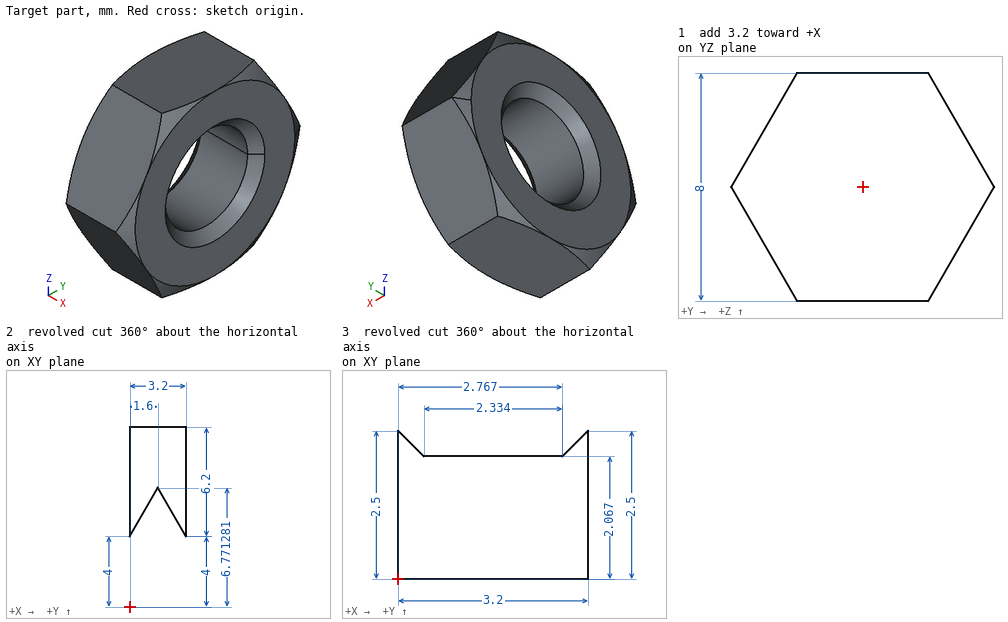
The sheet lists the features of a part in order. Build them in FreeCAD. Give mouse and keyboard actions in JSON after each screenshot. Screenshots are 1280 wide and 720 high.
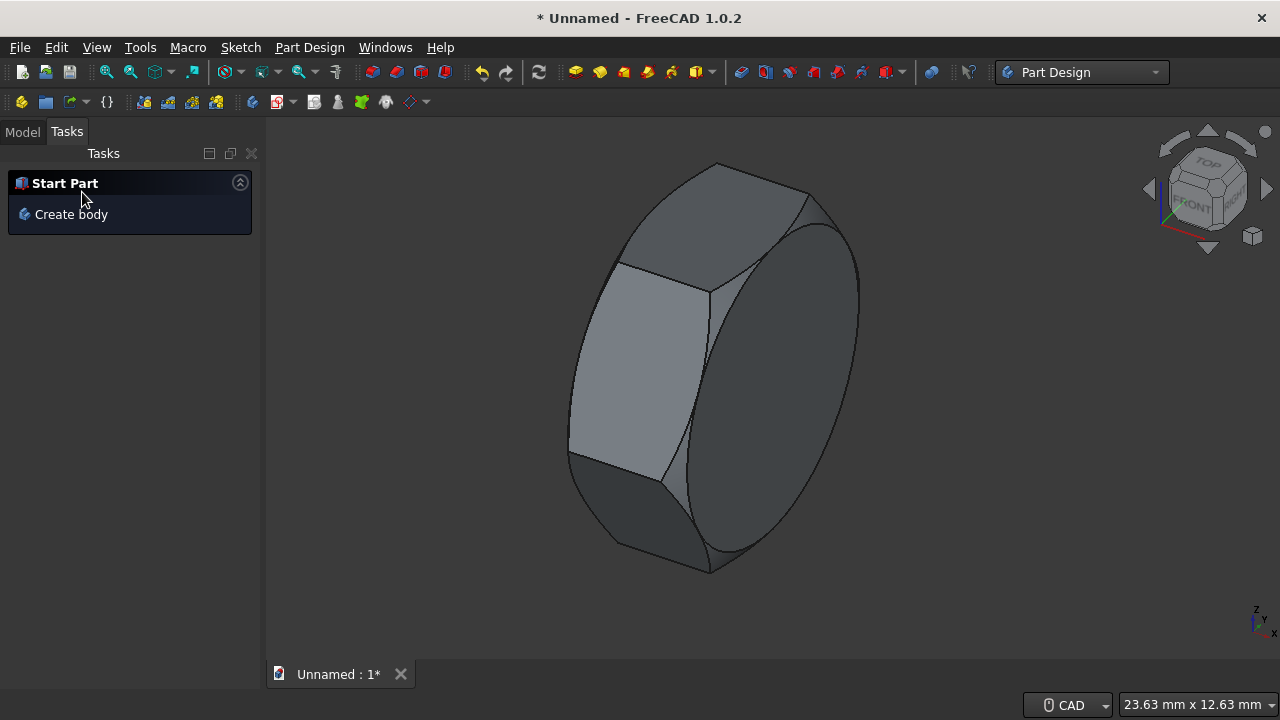
{"action": "key", "text": "v f"}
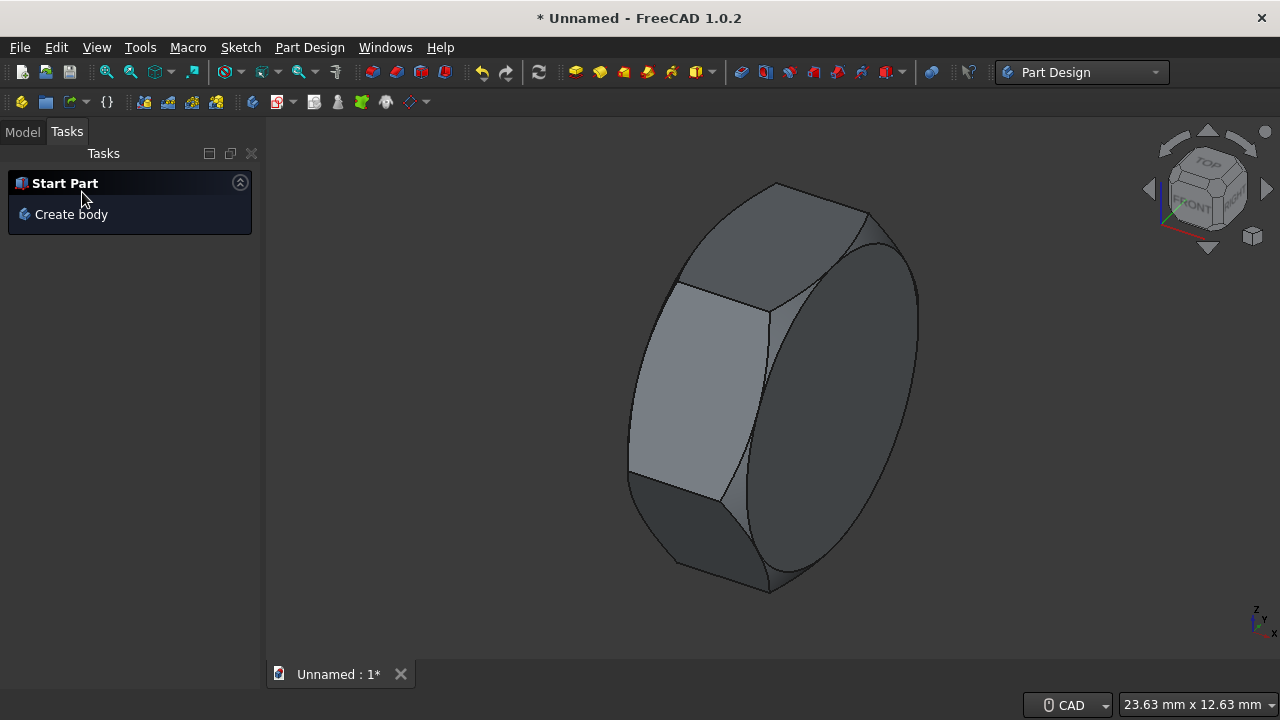
{"action": "left_click", "coordinate": [278, 102]}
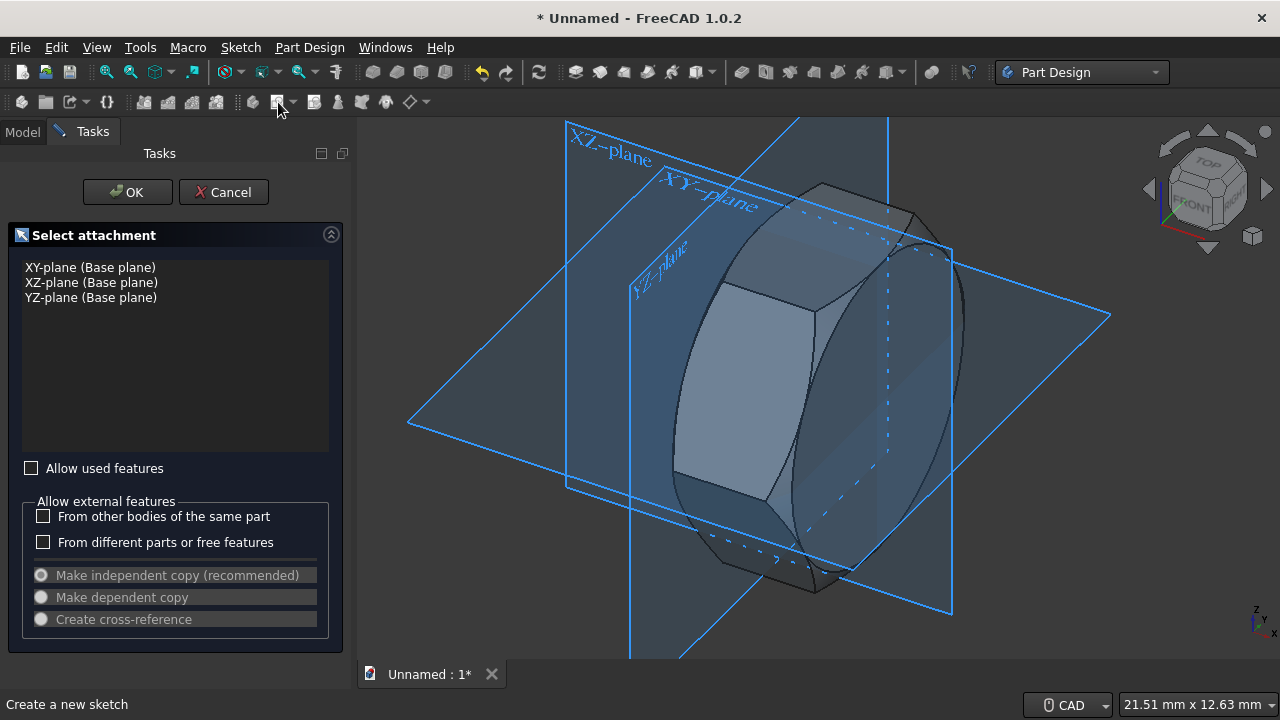
{"action": "left_click", "coordinate": [82, 268]}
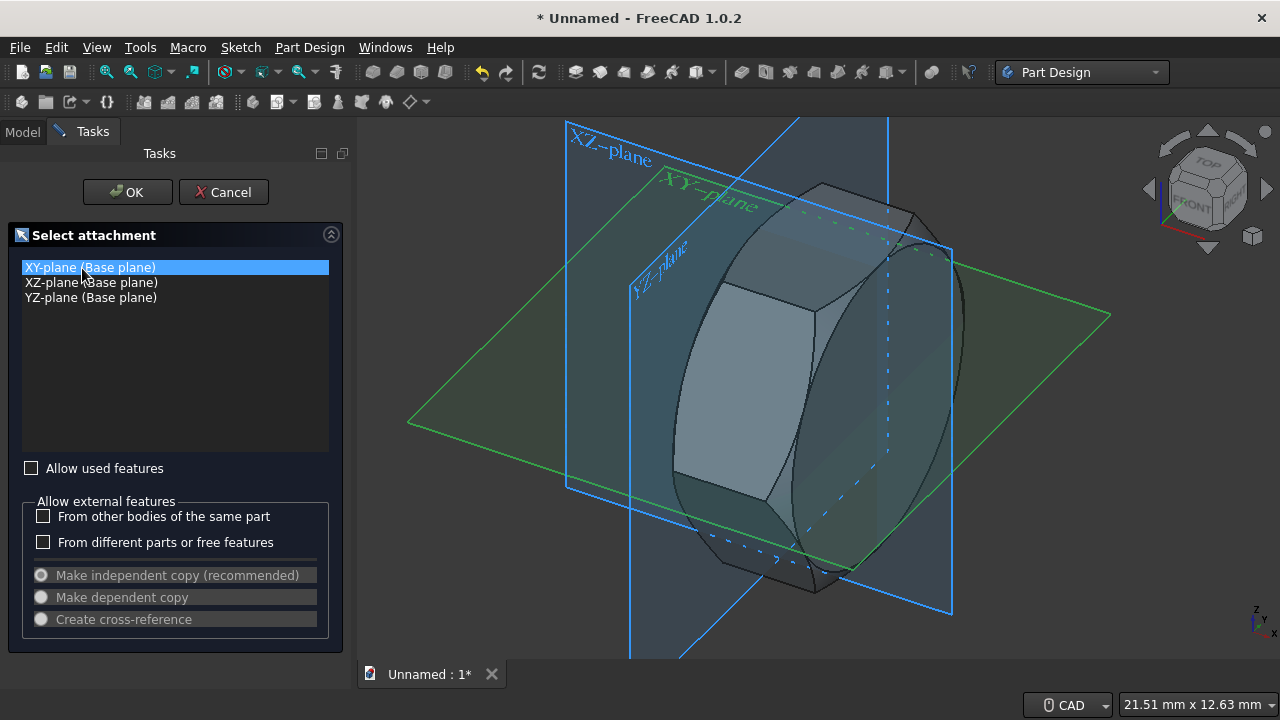
{"action": "left_click", "coordinate": [128, 192]}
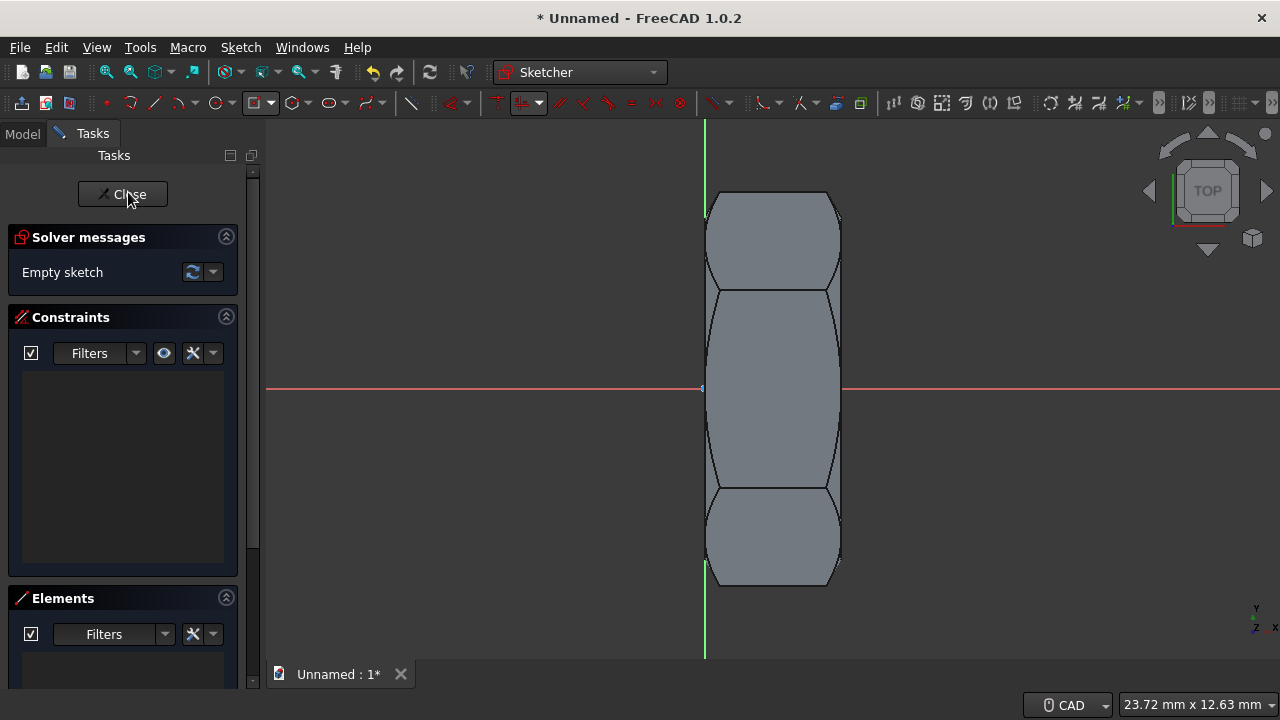
{"action": "key", "text": "q s"}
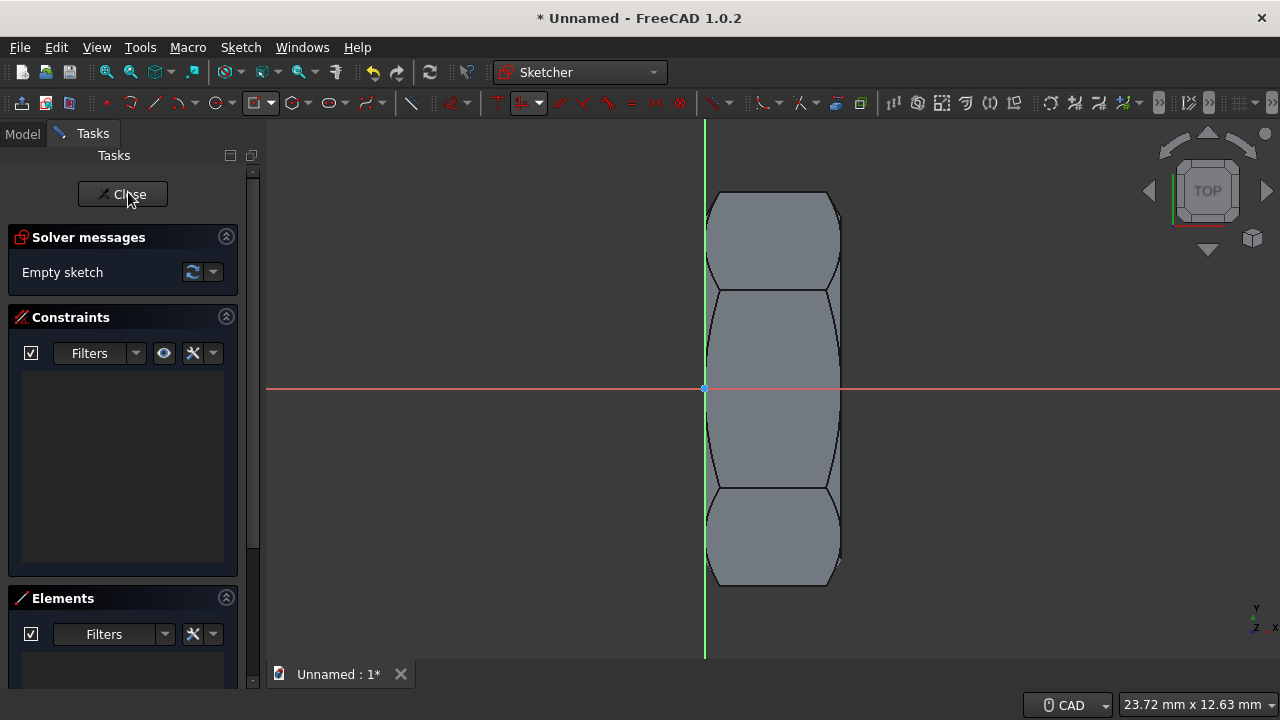
{"action": "scroll", "coordinate": [803, 313], "scroll_direction": "up", "scroll_amount": 6}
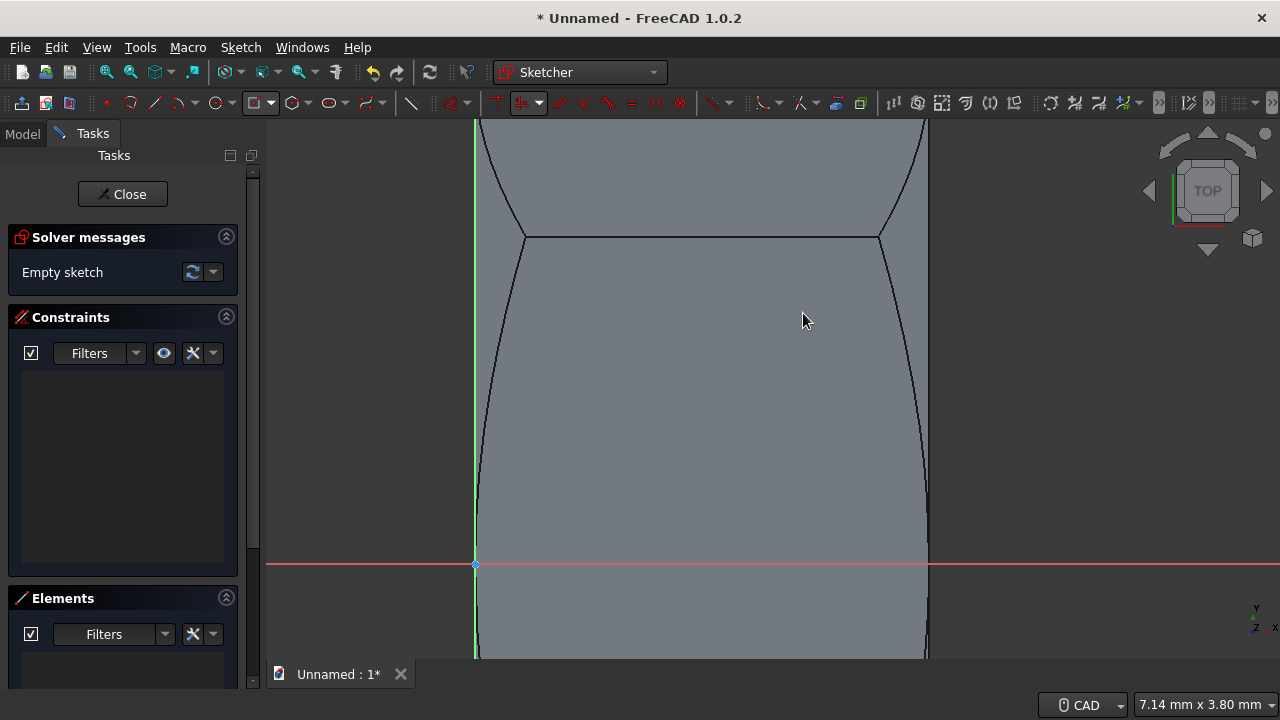
{"action": "key", "text": "g m"}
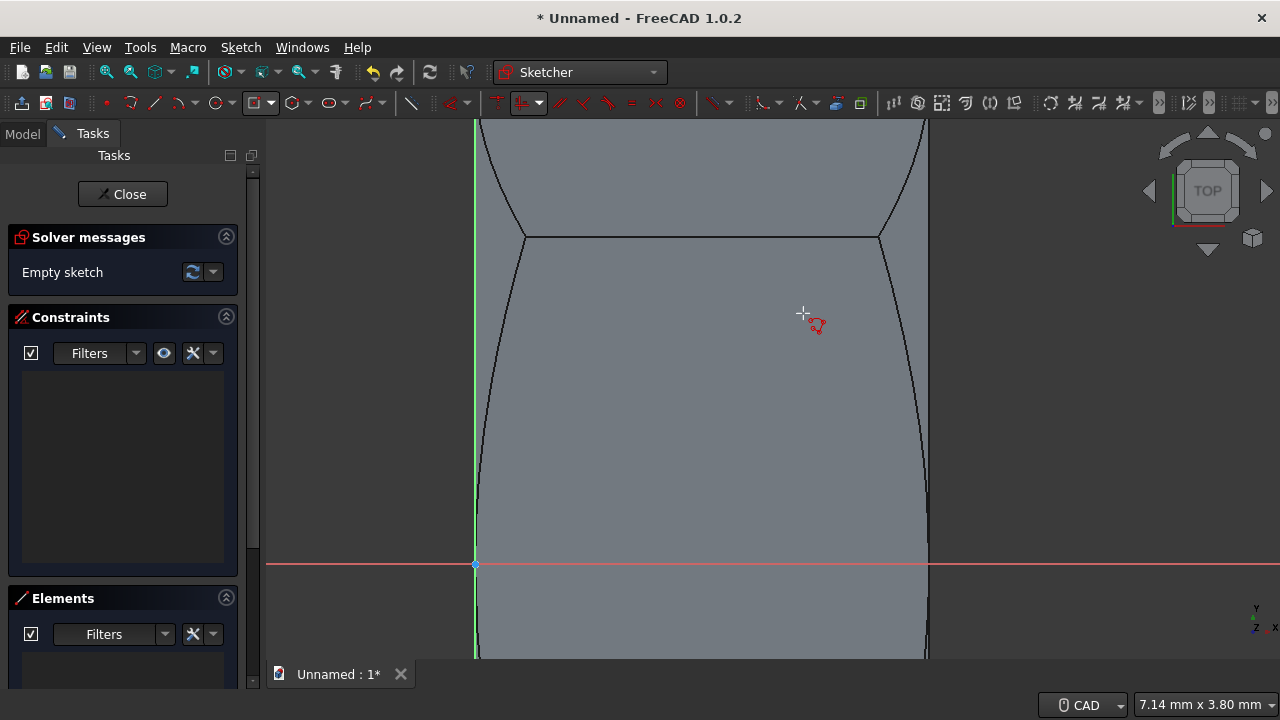
{"action": "left_click", "coordinate": [475, 564]}
{"action": "left_click", "coordinate": [929, 555]}
{"action": "left_click", "coordinate": [929, 210]}
{"action": "left_click", "coordinate": [868, 271]}
{"action": "left_click", "coordinate": [537, 271]}
{"action": "left_click", "coordinate": [484, 210]}
{"action": "left_click", "coordinate": [475, 564]}
{"action": "key", "text": "Escape"}
{"action": "key", "text": "Escape"}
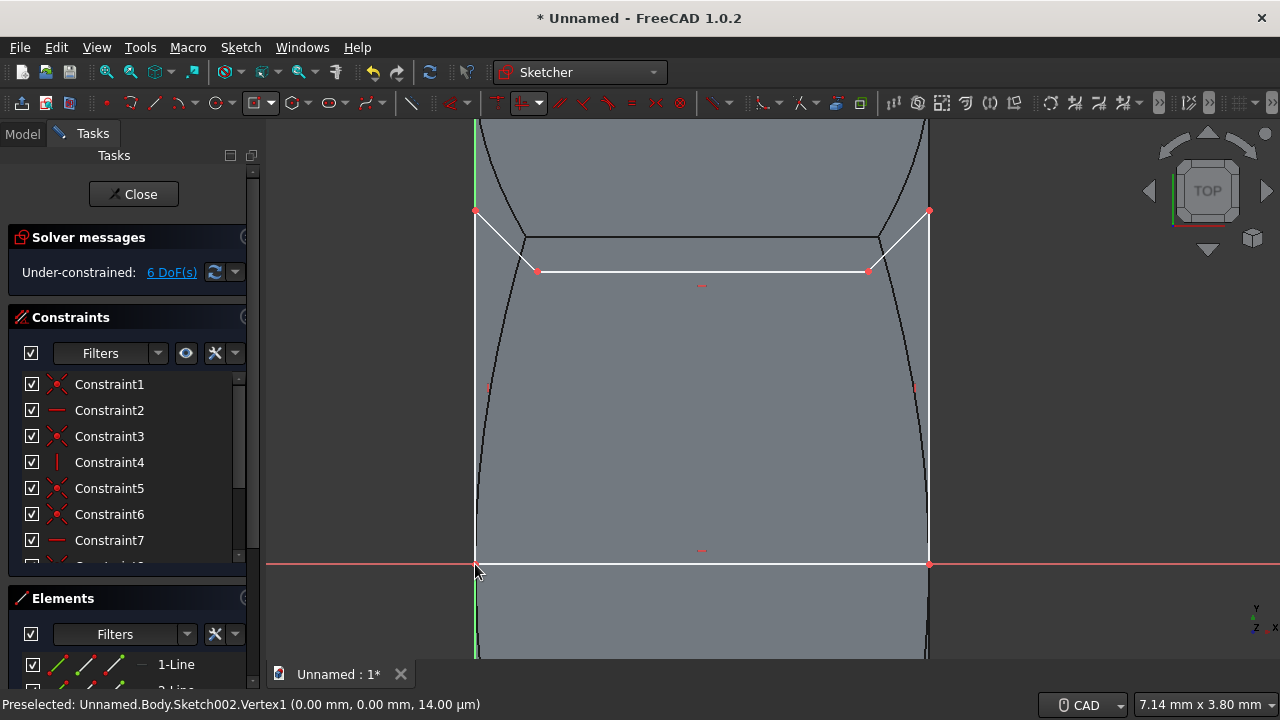
{"action": "key", "text": "d"}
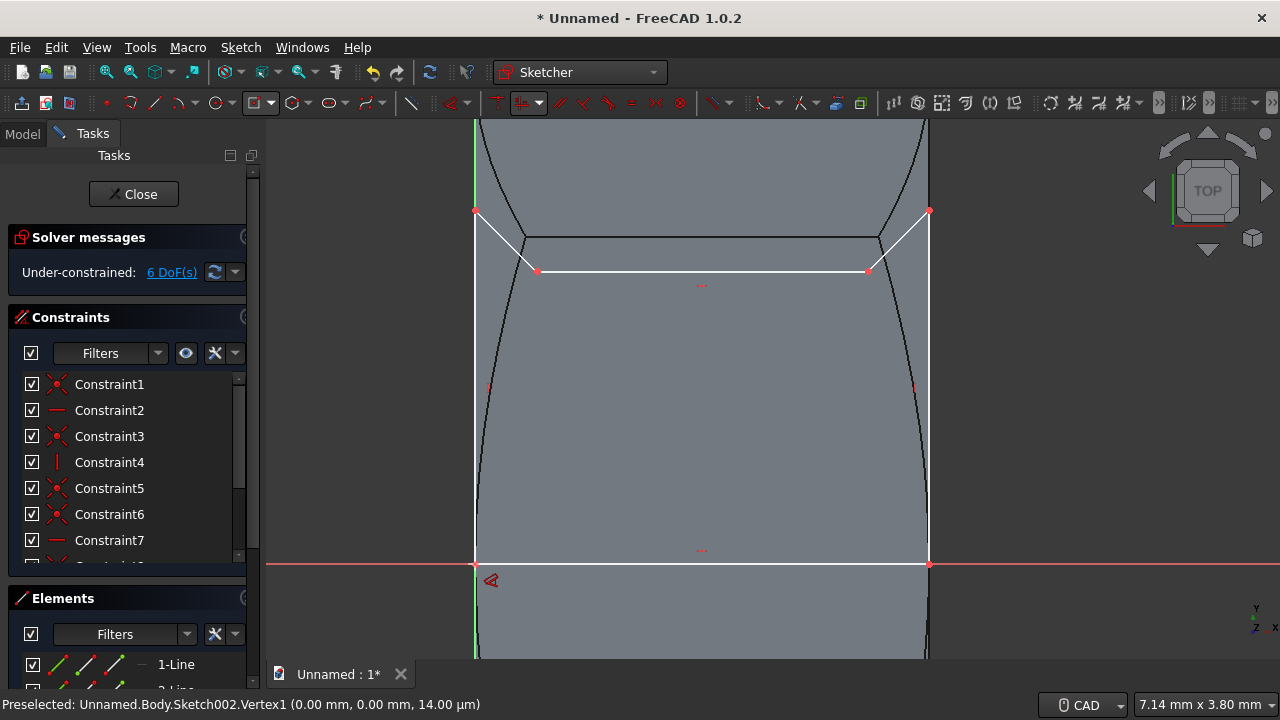
{"action": "left_click", "coordinate": [611, 564]}
{"action": "left_click", "coordinate": [702, 598]}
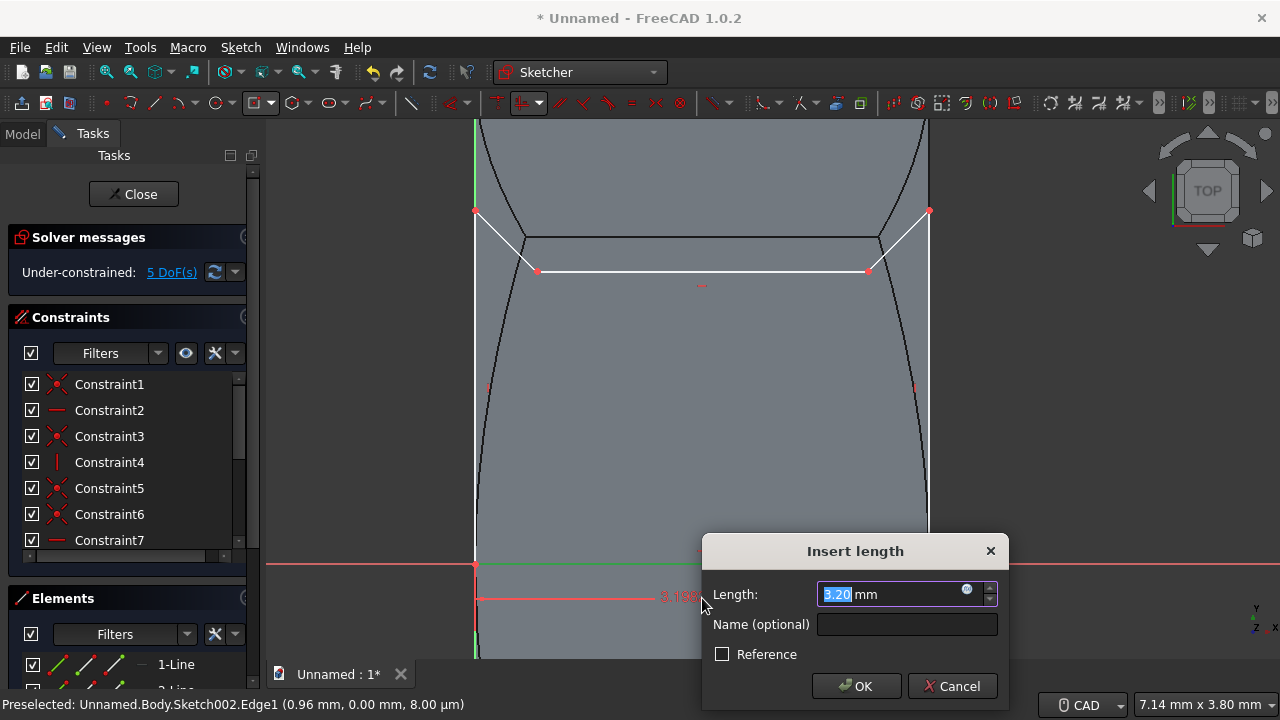
{"action": "type", "text": "3.2"}
{"action": "key", "text": "Return"}